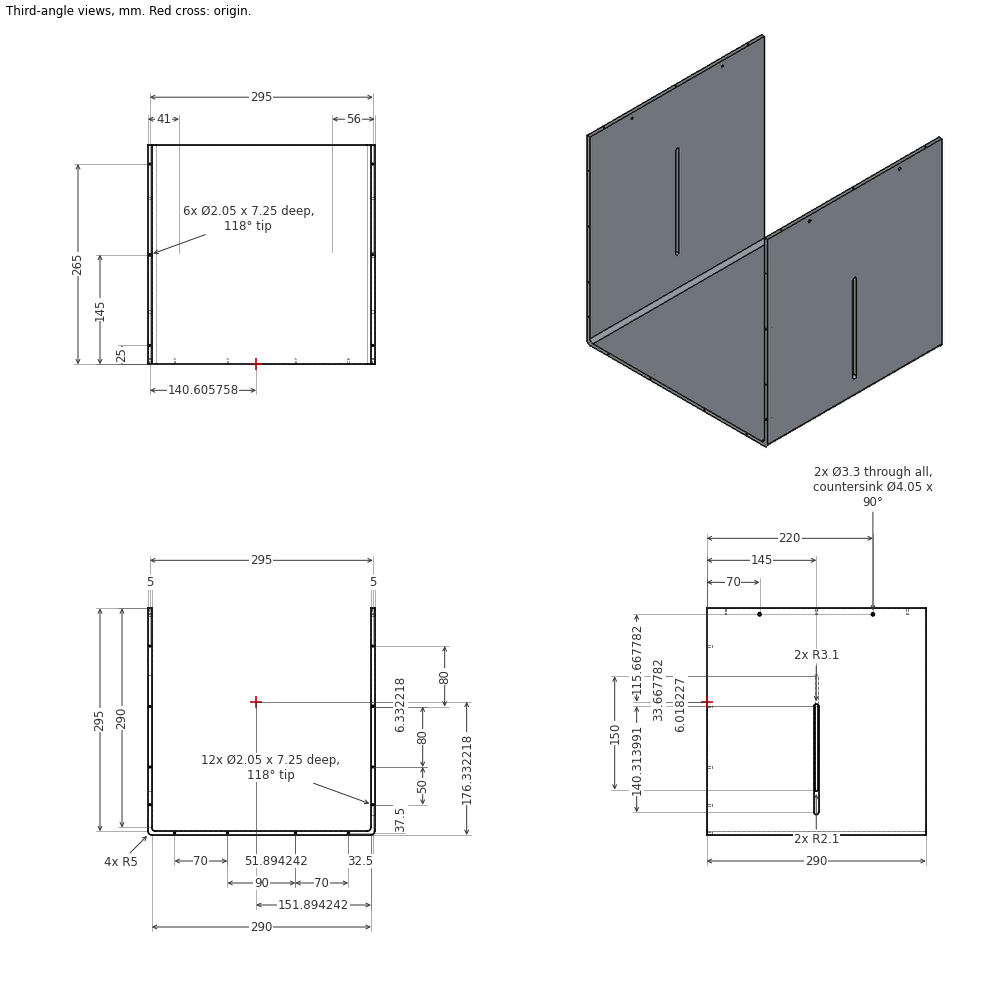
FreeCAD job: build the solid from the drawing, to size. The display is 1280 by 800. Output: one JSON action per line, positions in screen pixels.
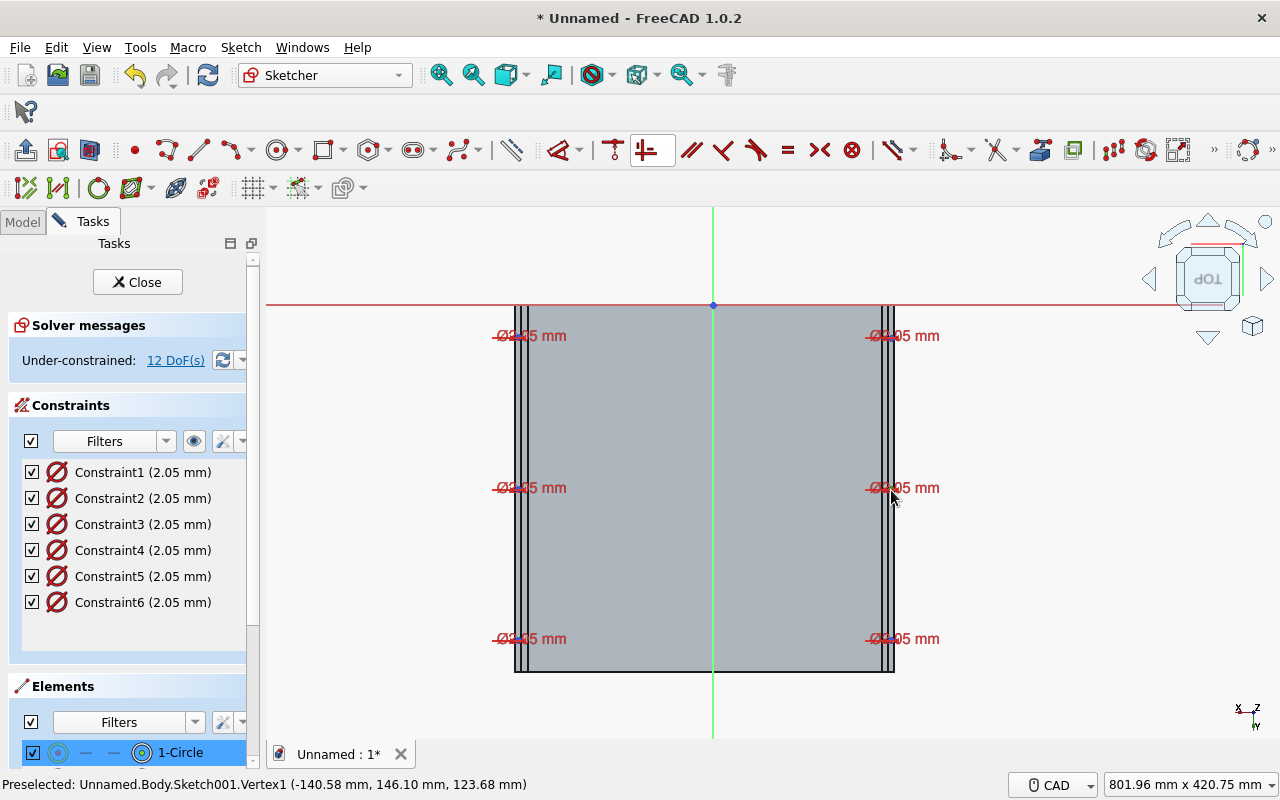
{"action": "left_click", "coordinate": [891, 641]}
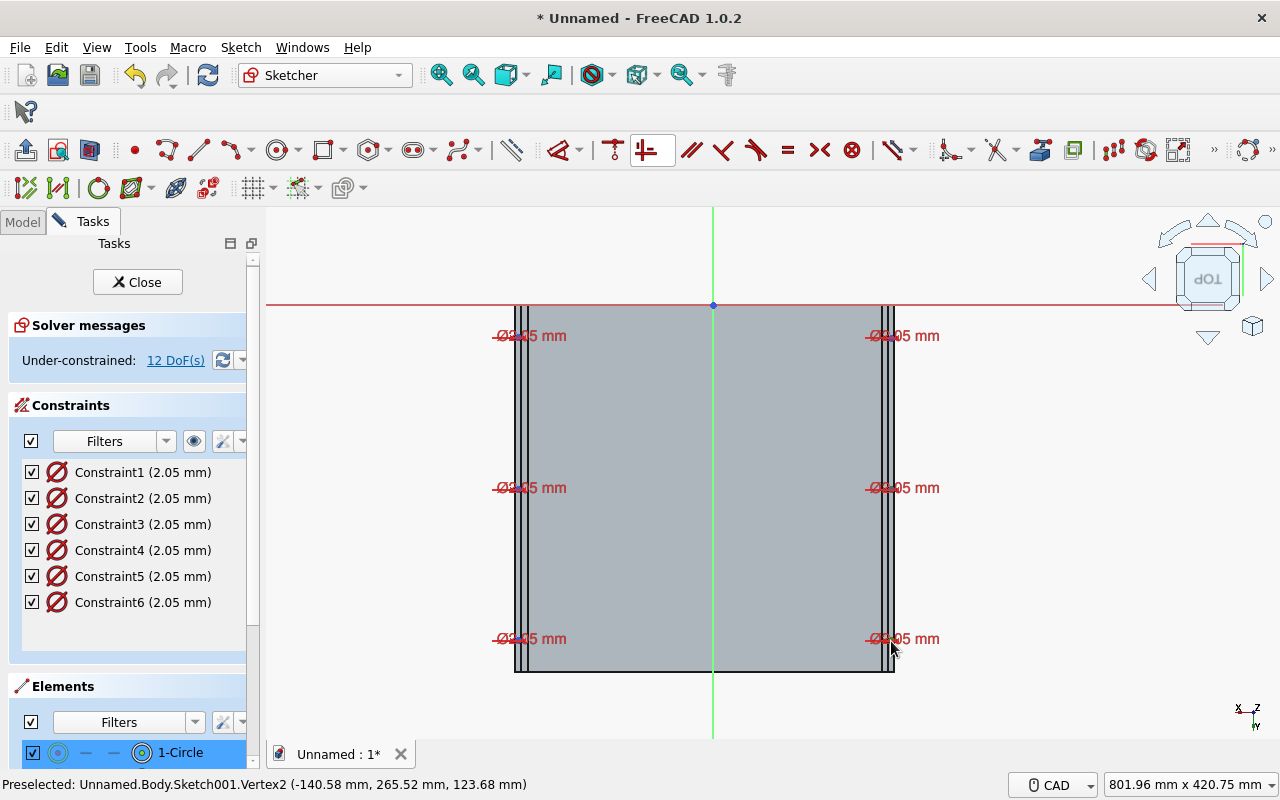
{"action": "key", "text": "v"}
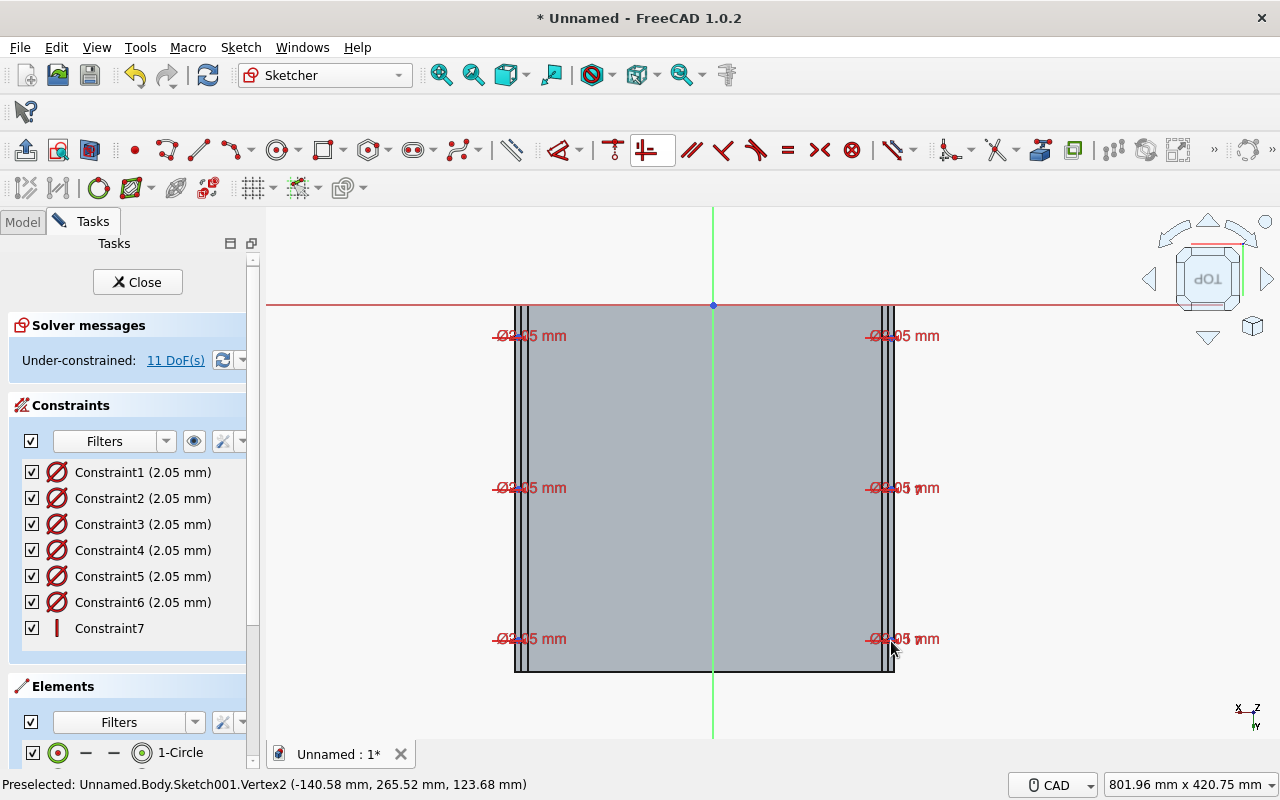
{"action": "left_click", "coordinate": [891, 490]}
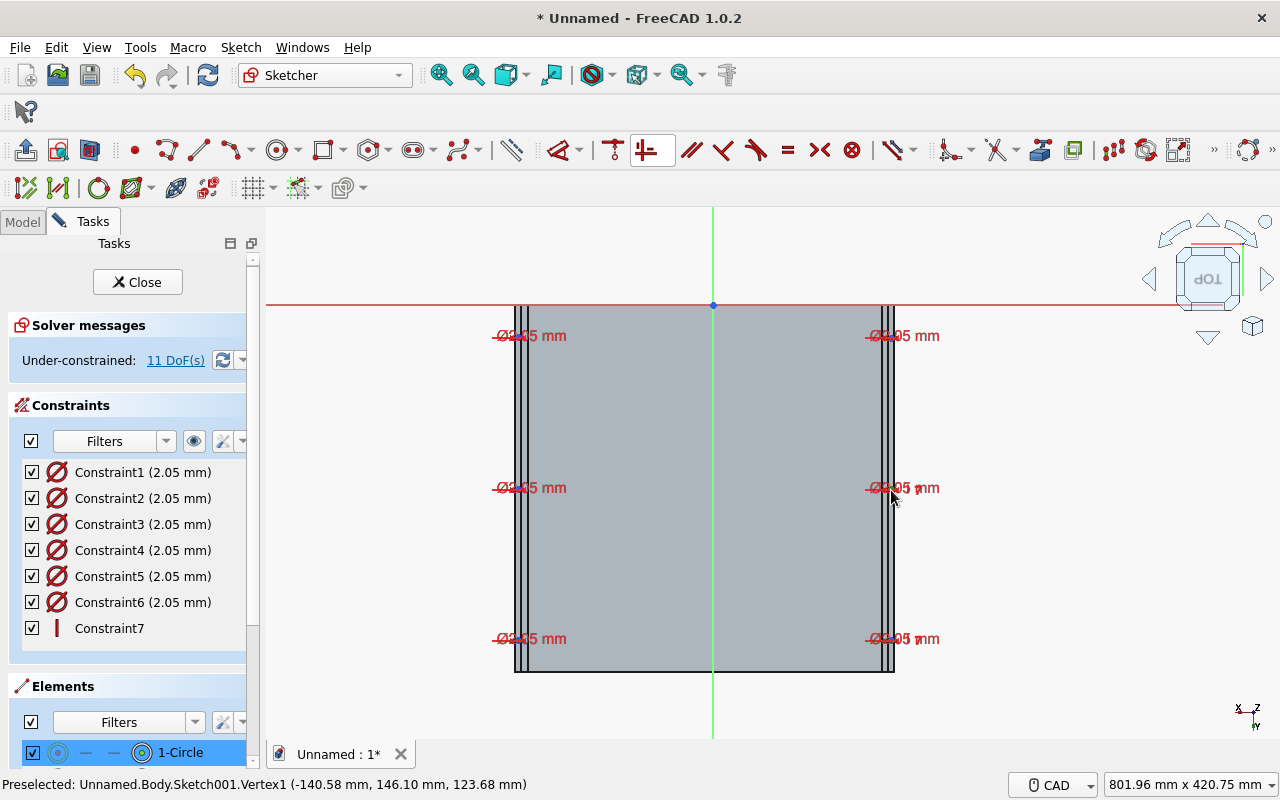
{"action": "left_click", "coordinate": [891, 338]}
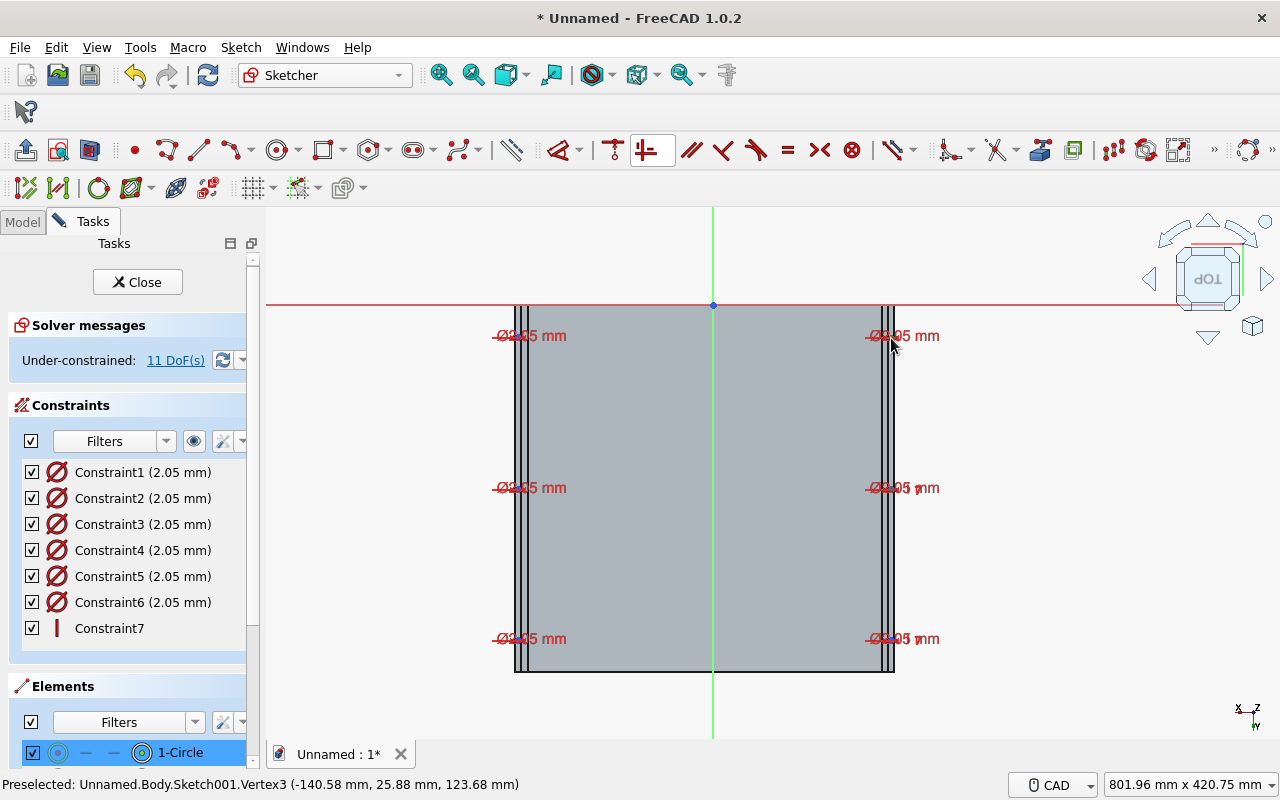
{"action": "left_click", "coordinate": [670, 150]}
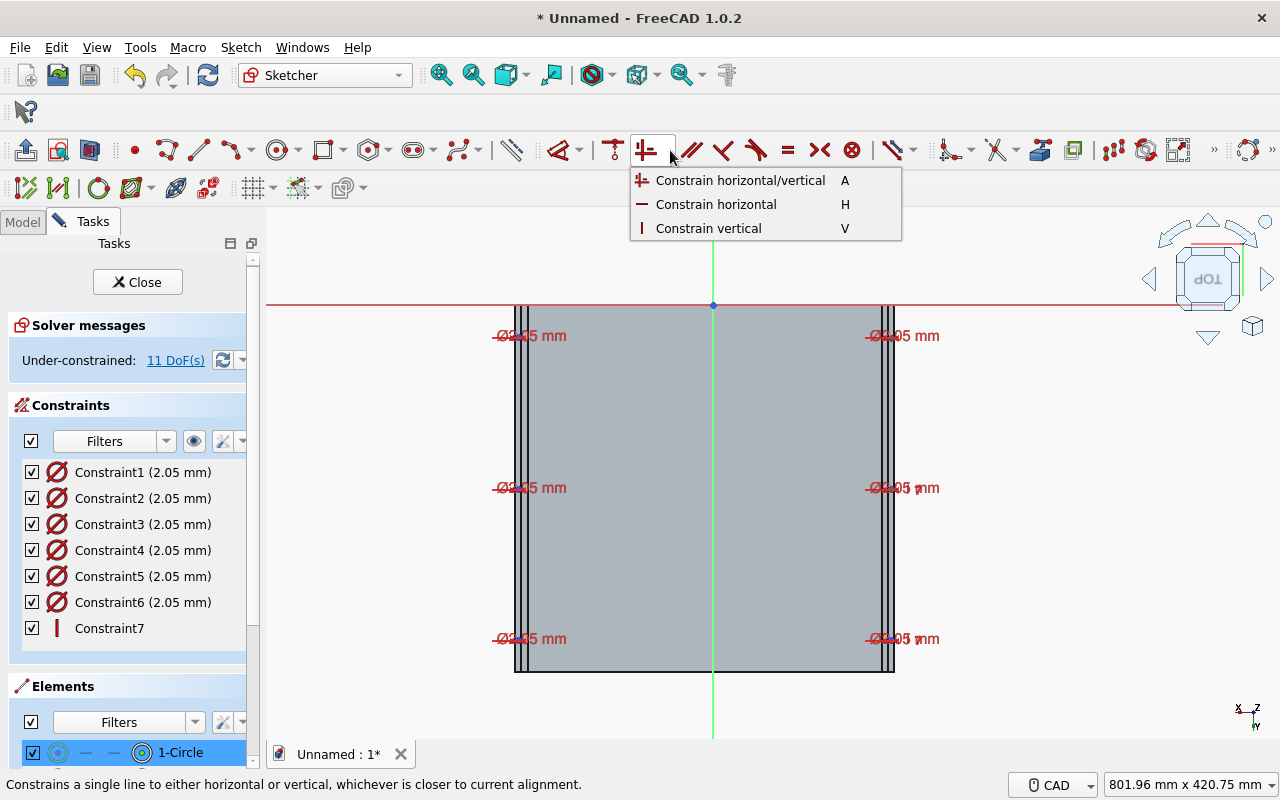
{"action": "left_click", "coordinate": [766, 228]}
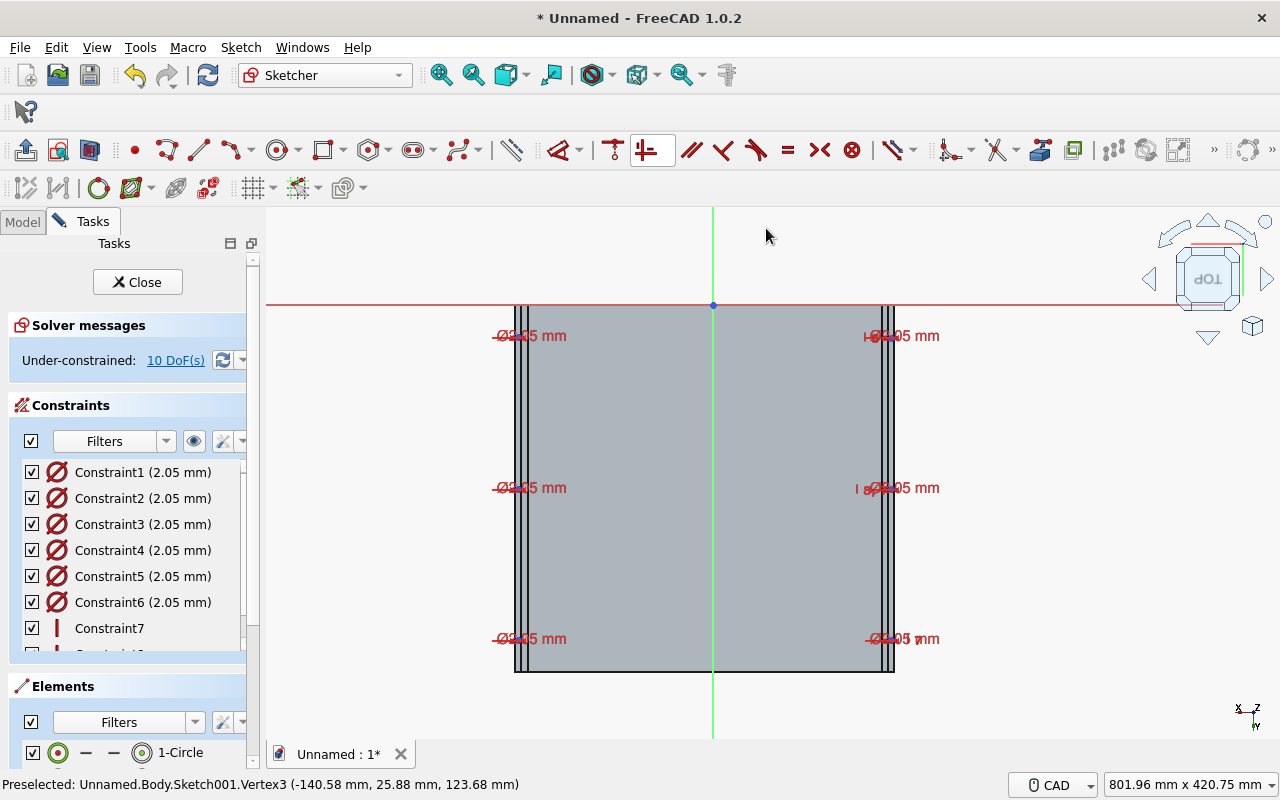
{"action": "left_click", "coordinate": [891, 490]}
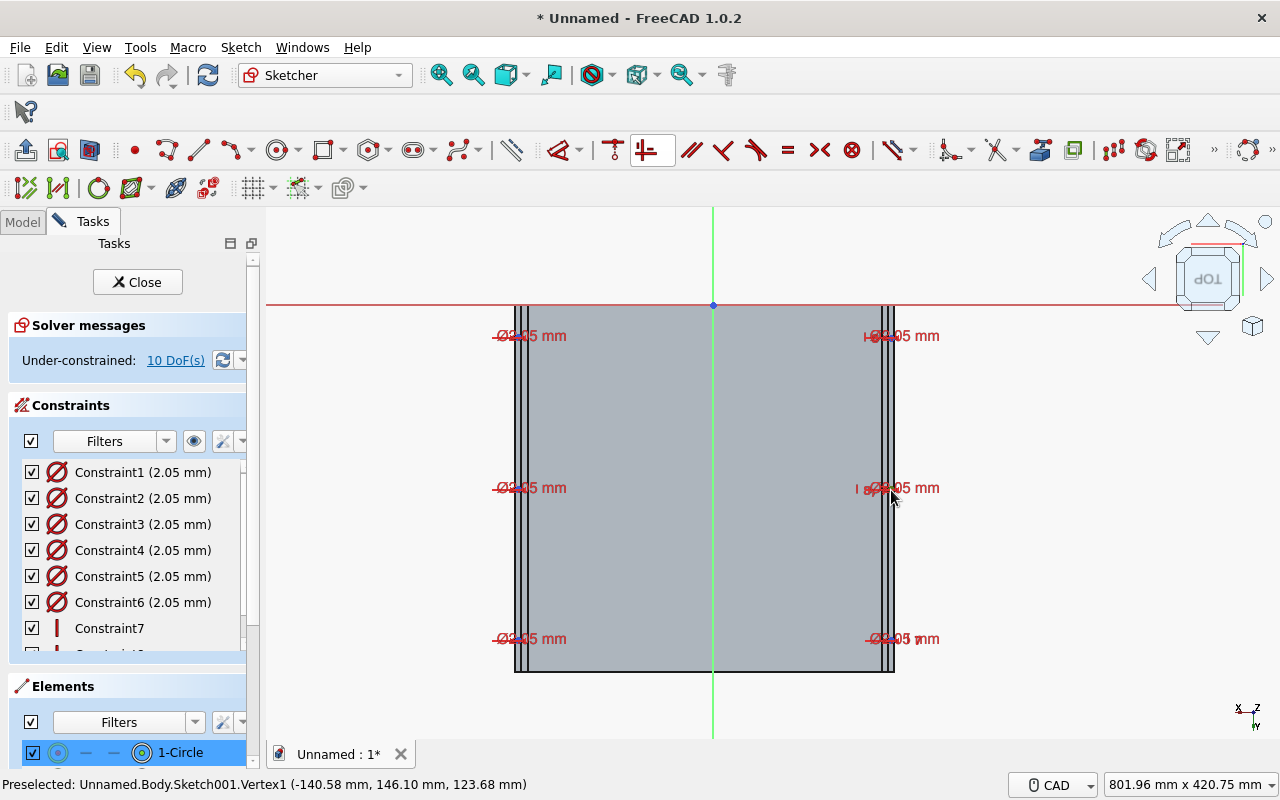
{"action": "left_click", "coordinate": [518, 490]}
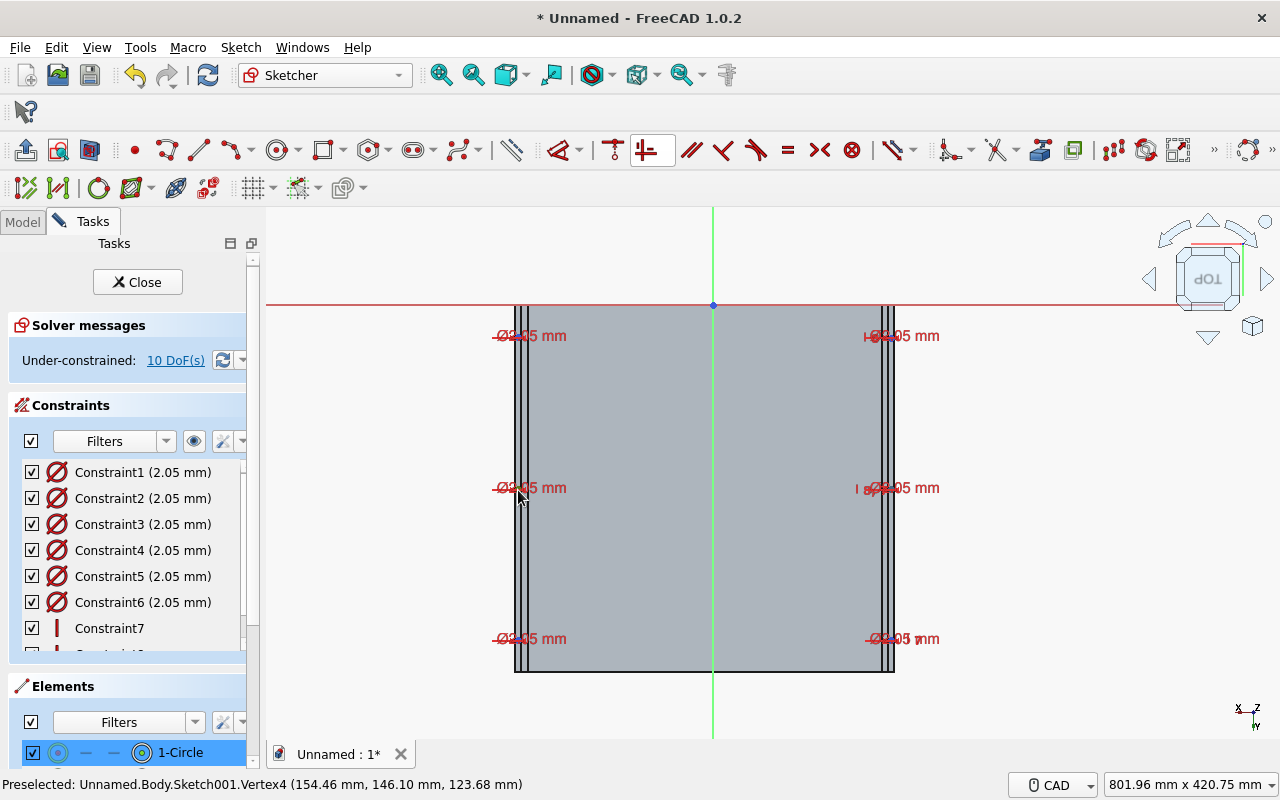
{"action": "left_click", "coordinate": [670, 150]}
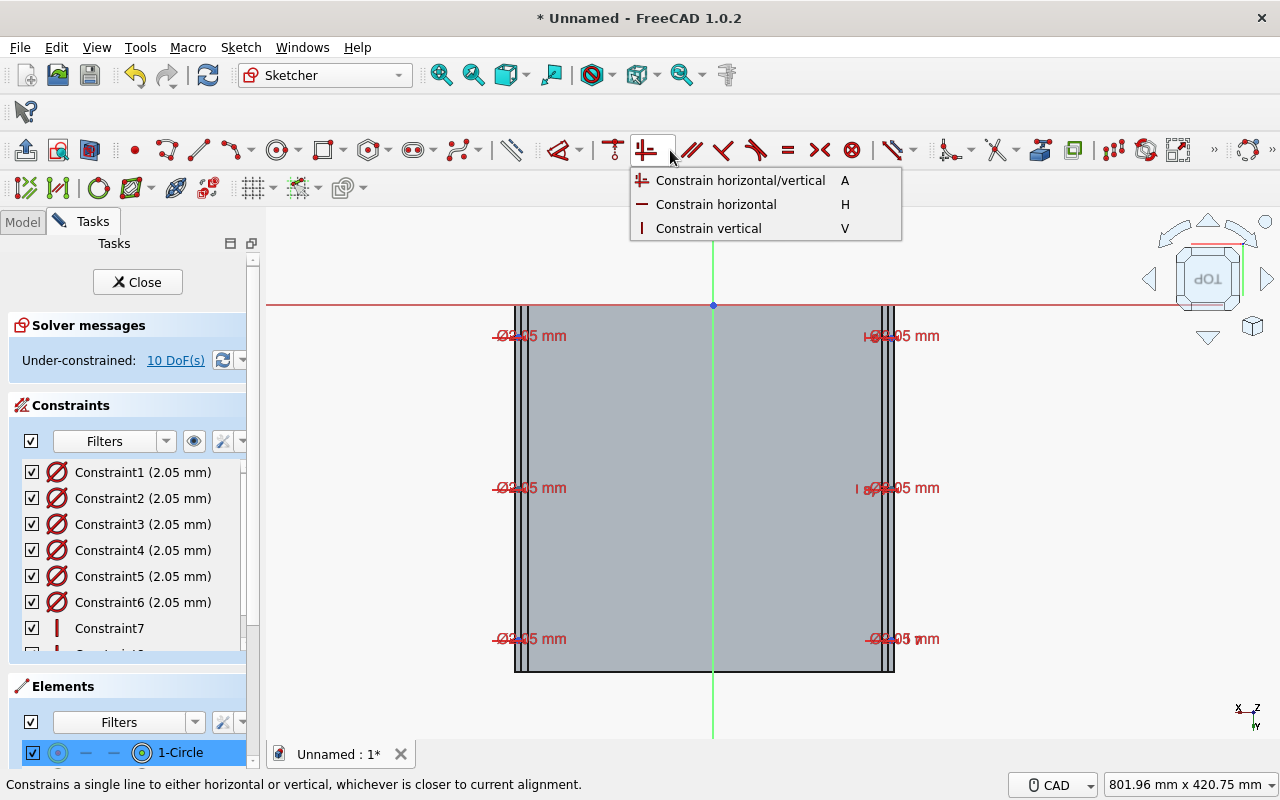
{"action": "left_click", "coordinate": [766, 204]}